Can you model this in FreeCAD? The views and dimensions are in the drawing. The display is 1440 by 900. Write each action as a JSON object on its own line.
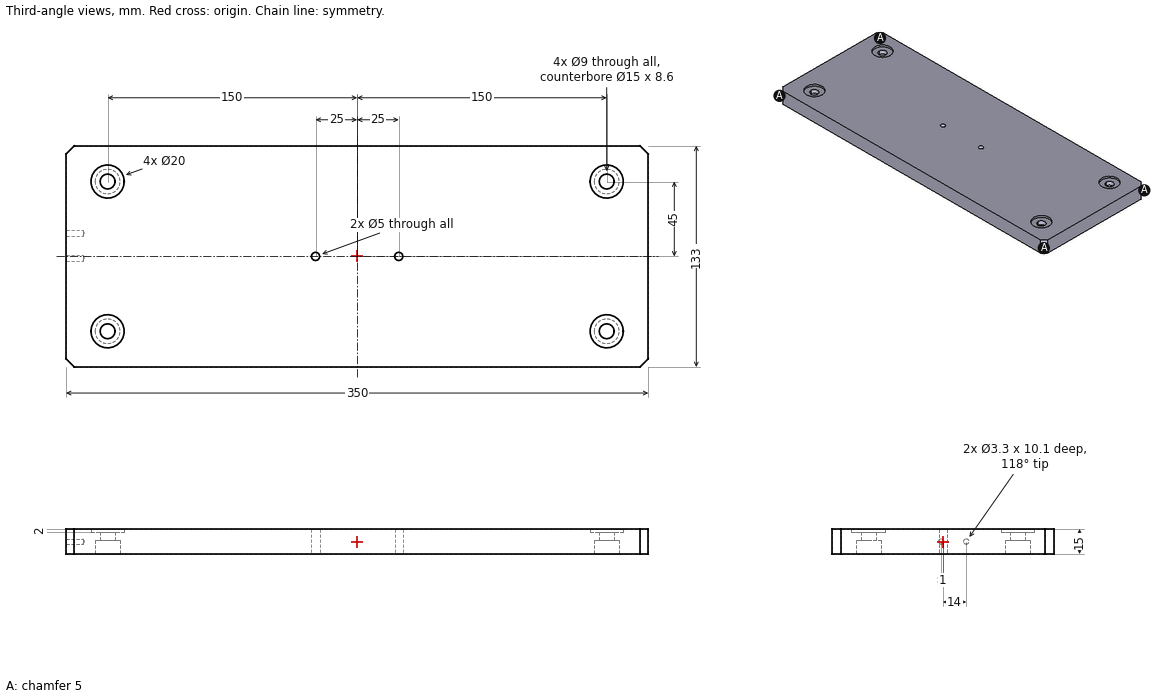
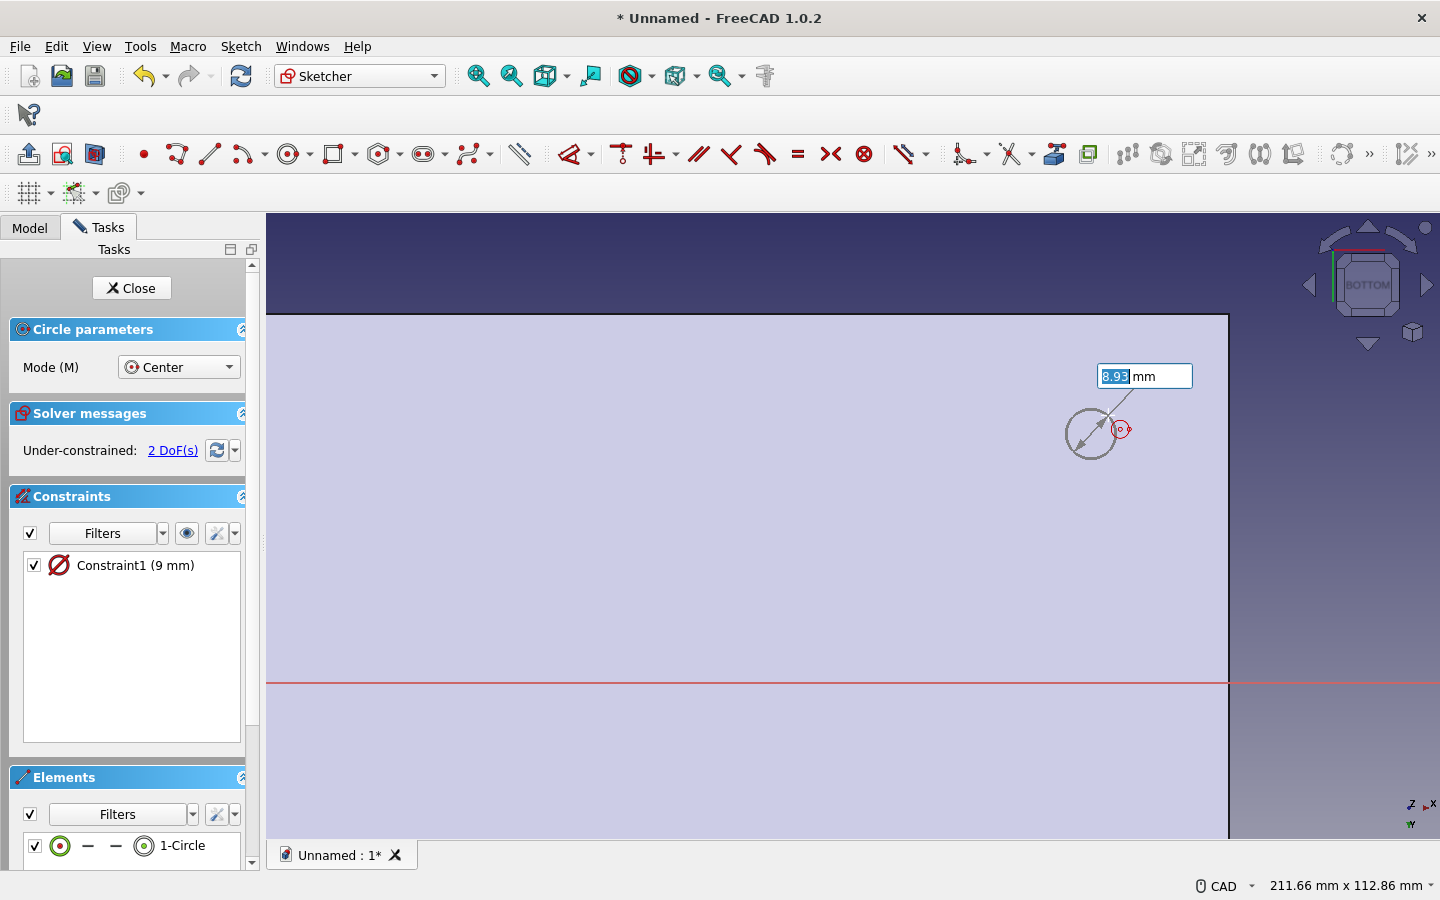
{"action": "type", "text": "9"}
{"action": "key", "text": "Return"}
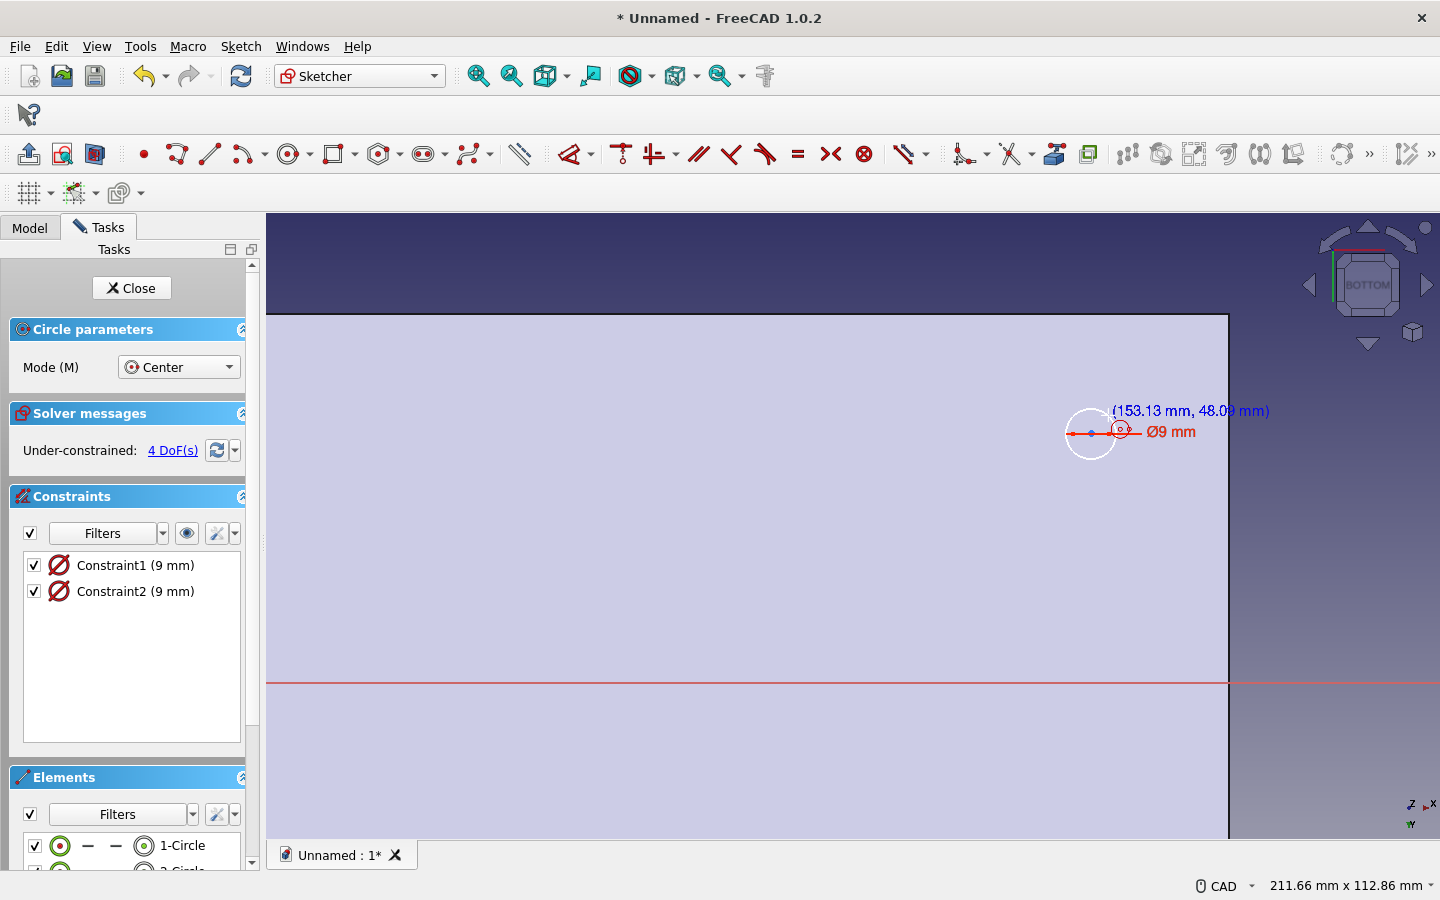
{"action": "scroll", "coordinate": [1091, 435], "scroll_direction": "down", "scroll_amount": 5}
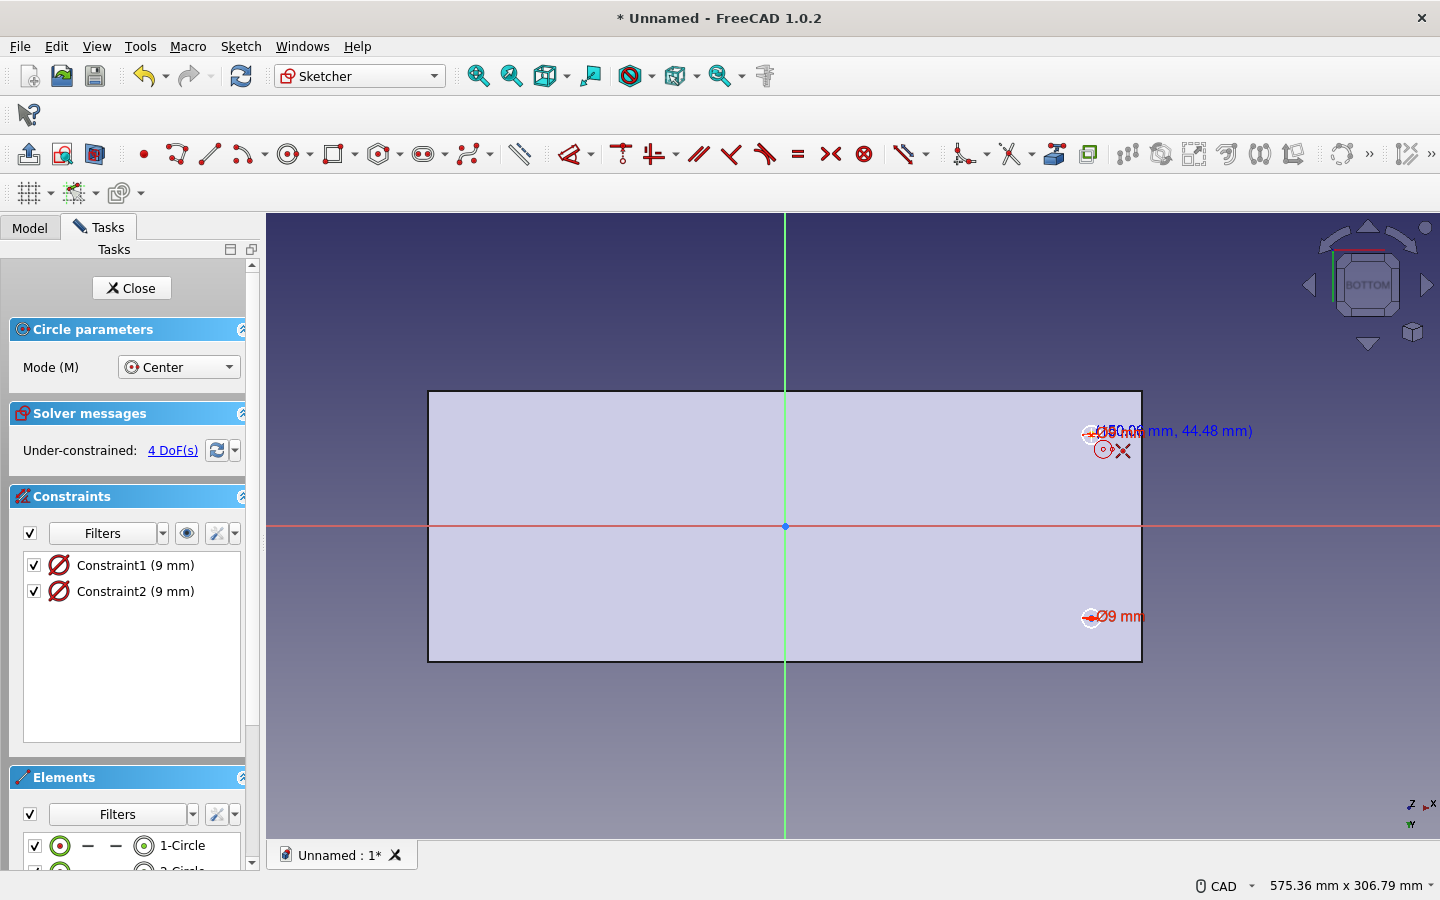
{"action": "scroll", "coordinate": [479, 435], "scroll_direction": "up", "scroll_amount": 5}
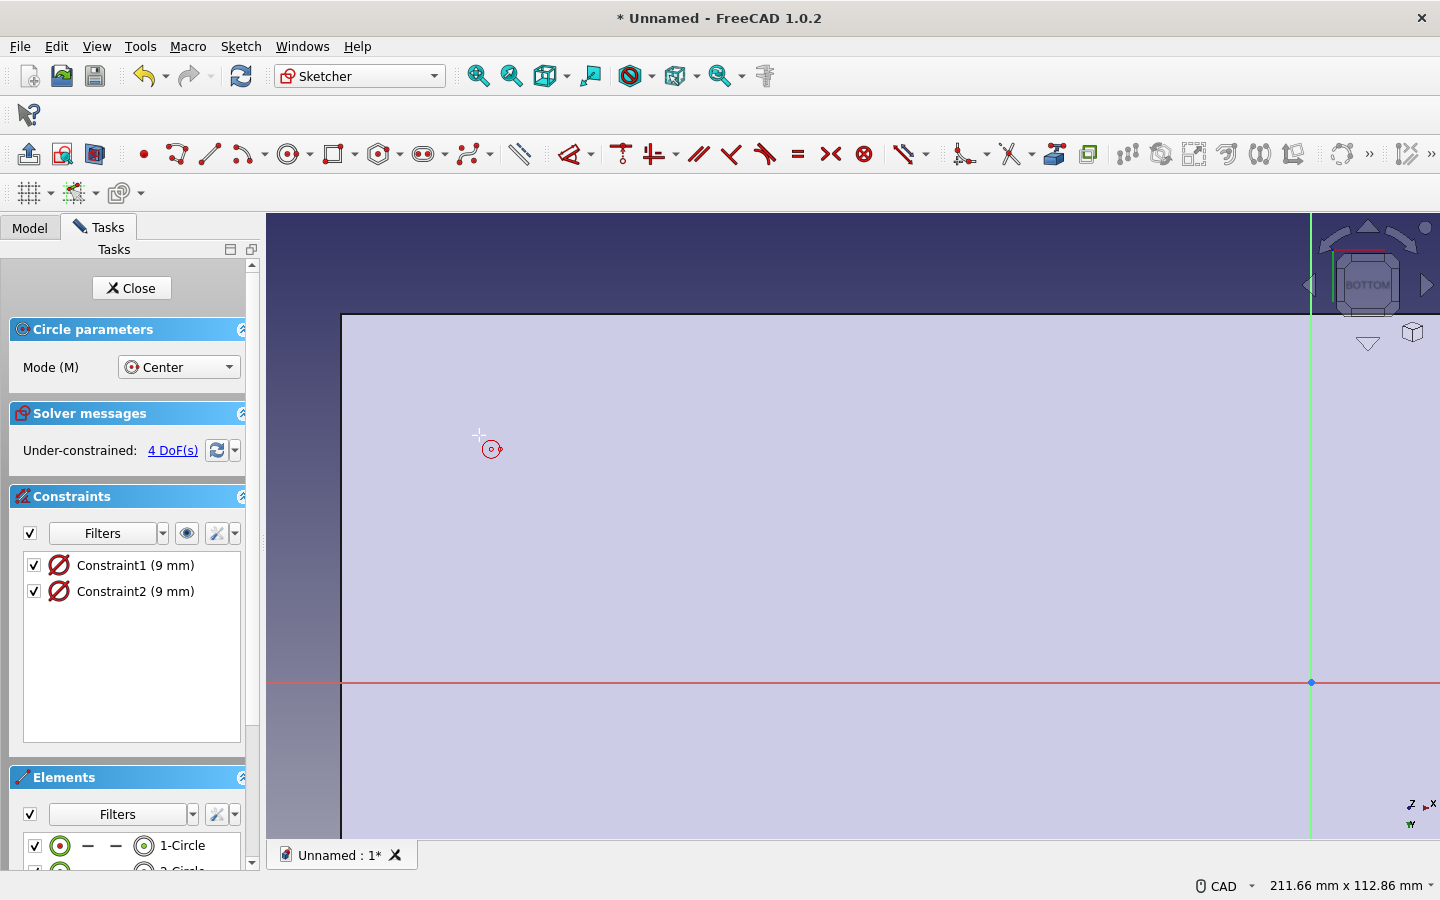
{"action": "left_click", "coordinate": [479, 433]}
{"action": "mouse_move", "coordinate": [497, 415]}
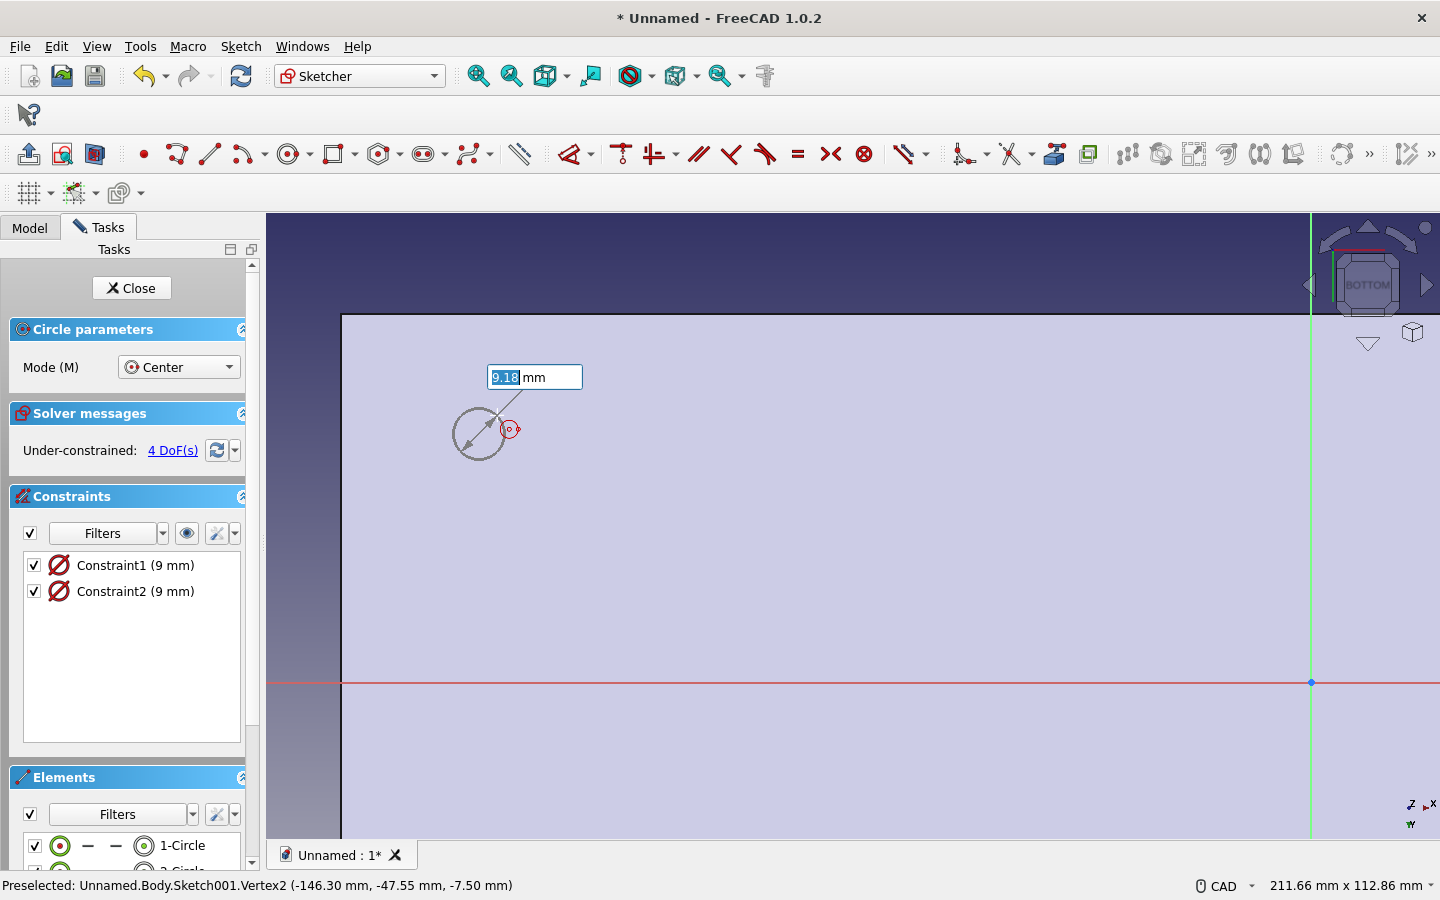
{"action": "type", "text": "9"}
{"action": "key", "text": "Return"}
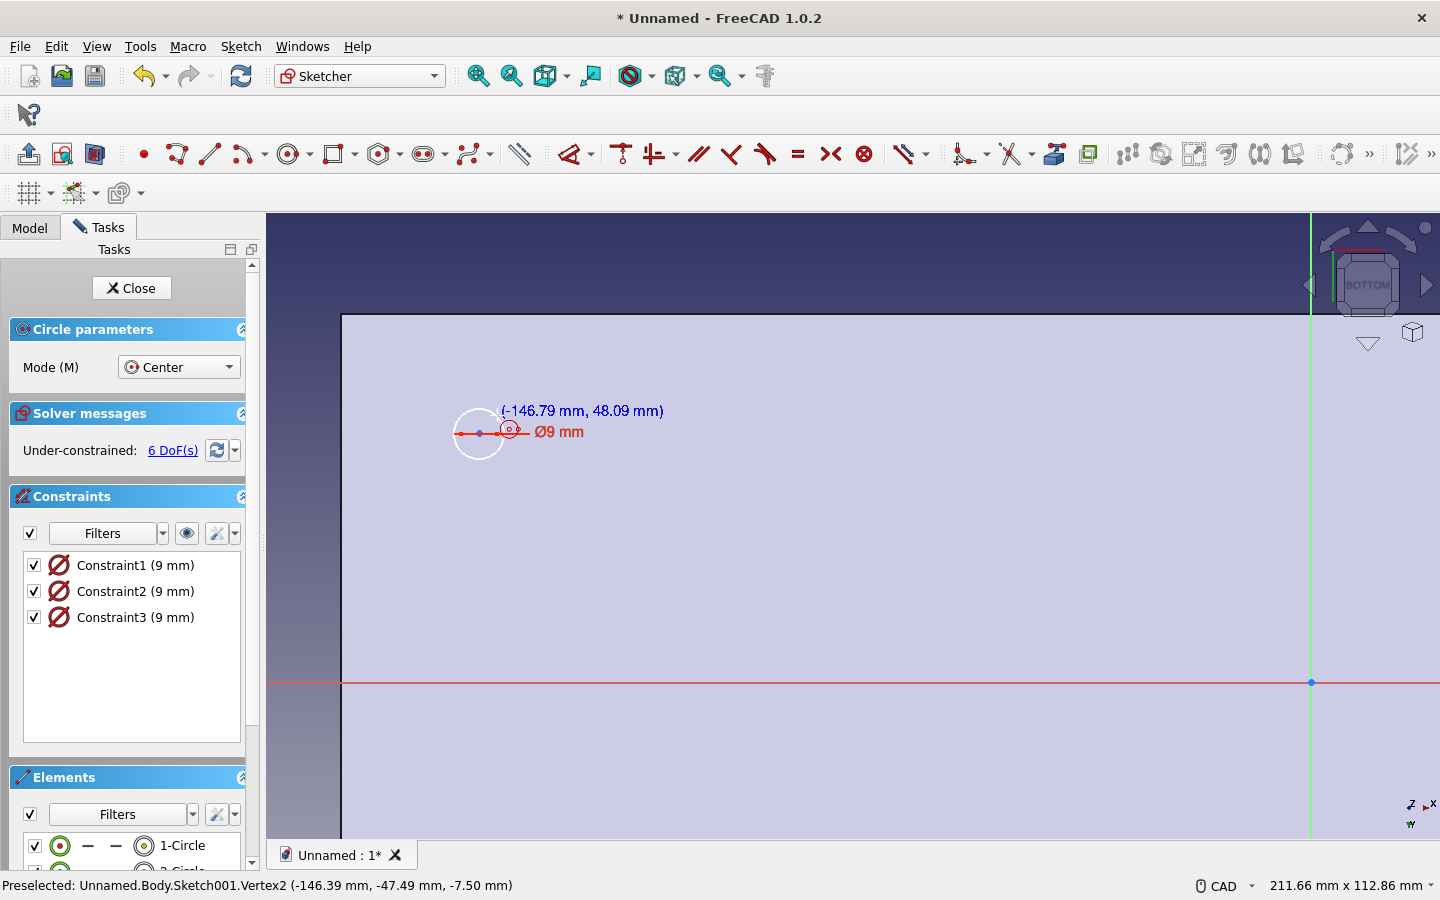
{"action": "scroll", "coordinate": [478, 435], "scroll_direction": "down", "scroll_amount": 5}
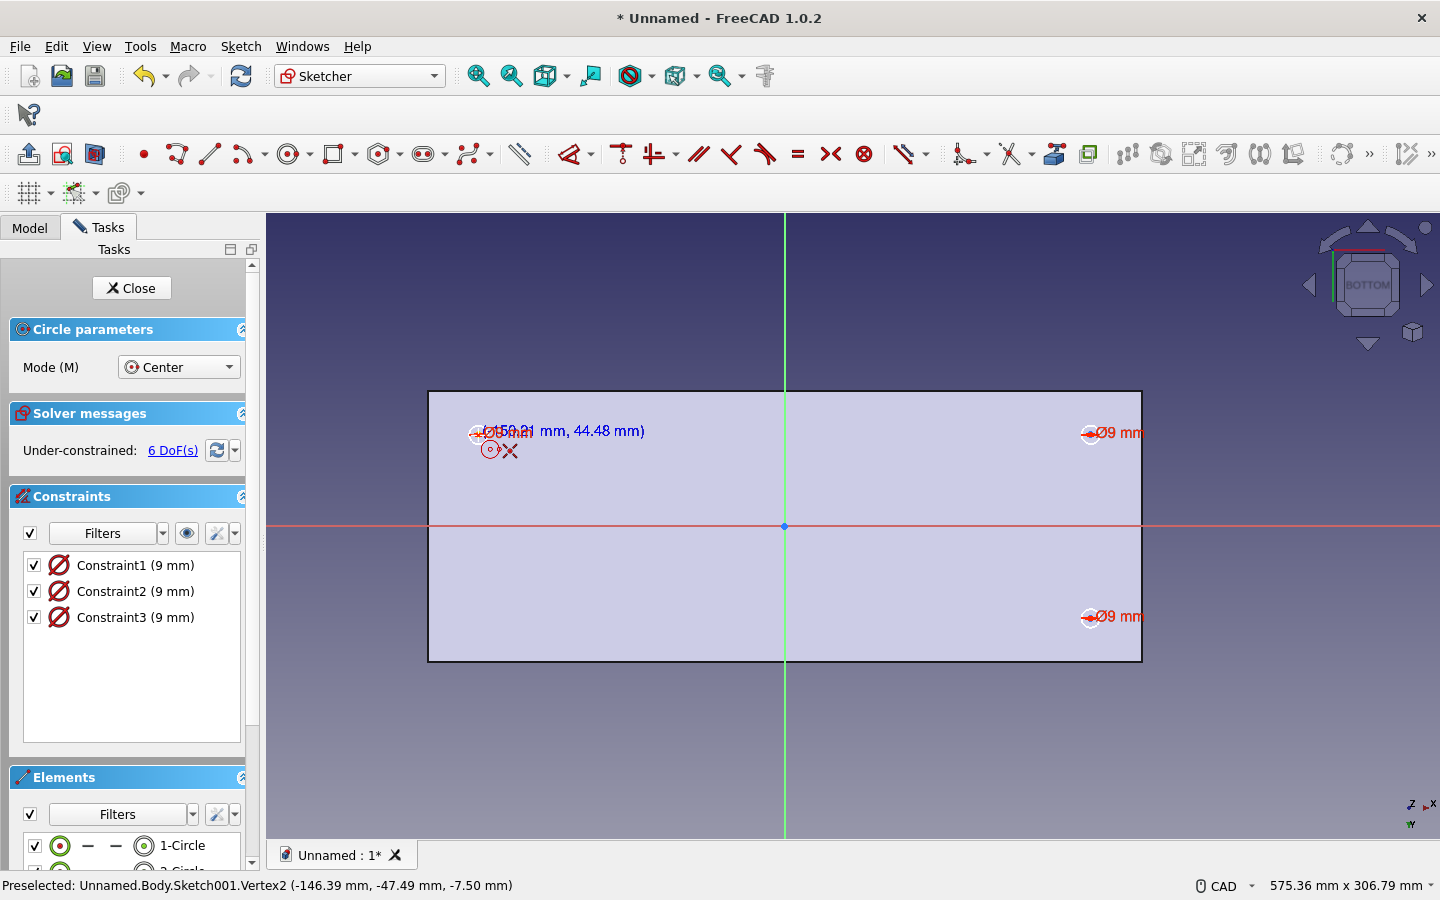
{"action": "scroll", "coordinate": [479, 618], "scroll_direction": "up", "scroll_amount": 5}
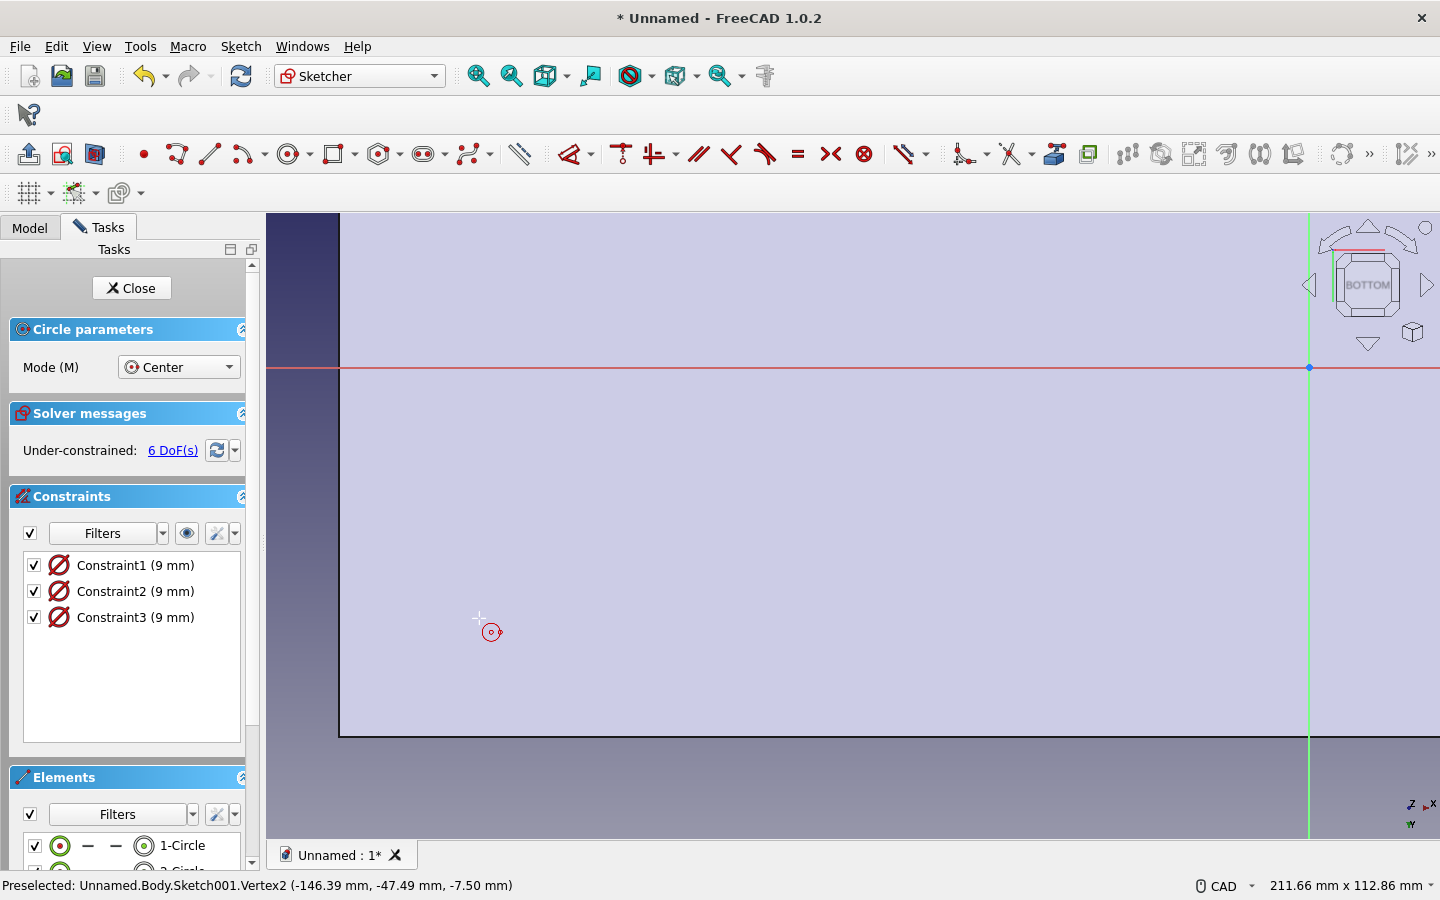
{"action": "left_click", "coordinate": [477, 617]}
{"action": "mouse_move", "coordinate": [495, 600]}